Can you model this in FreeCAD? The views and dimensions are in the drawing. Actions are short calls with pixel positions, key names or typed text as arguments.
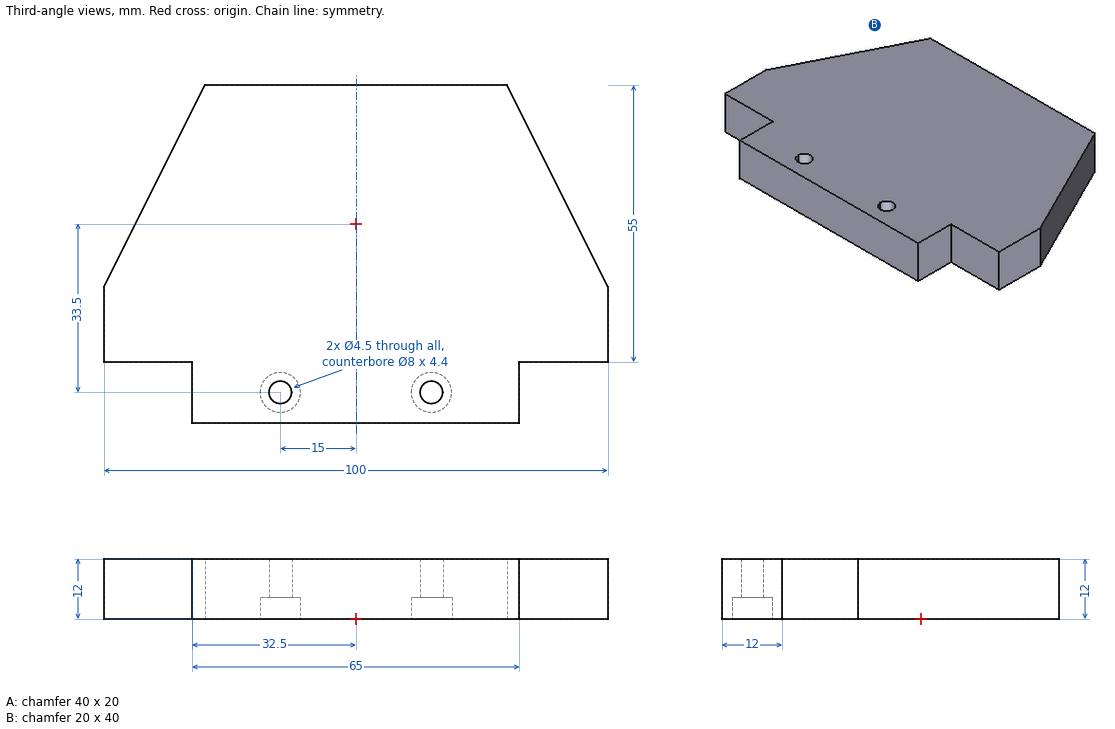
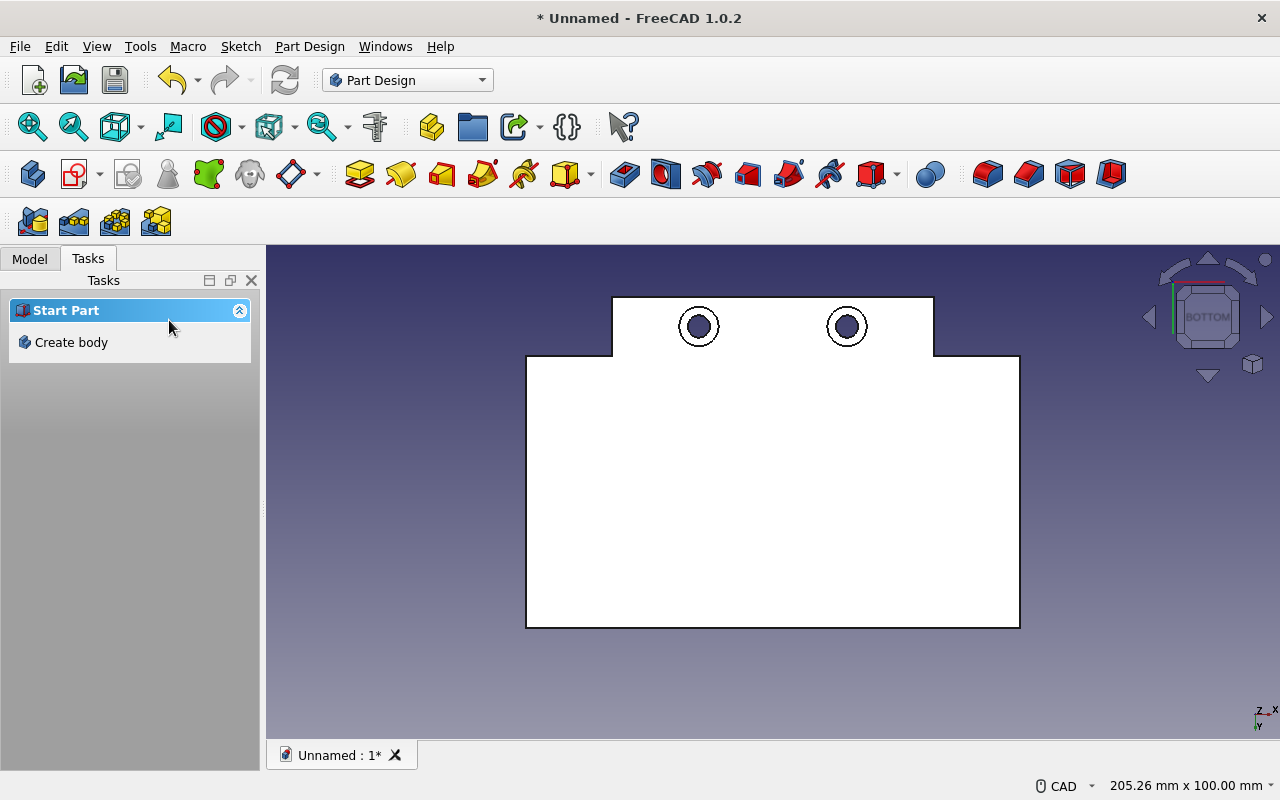
key(0)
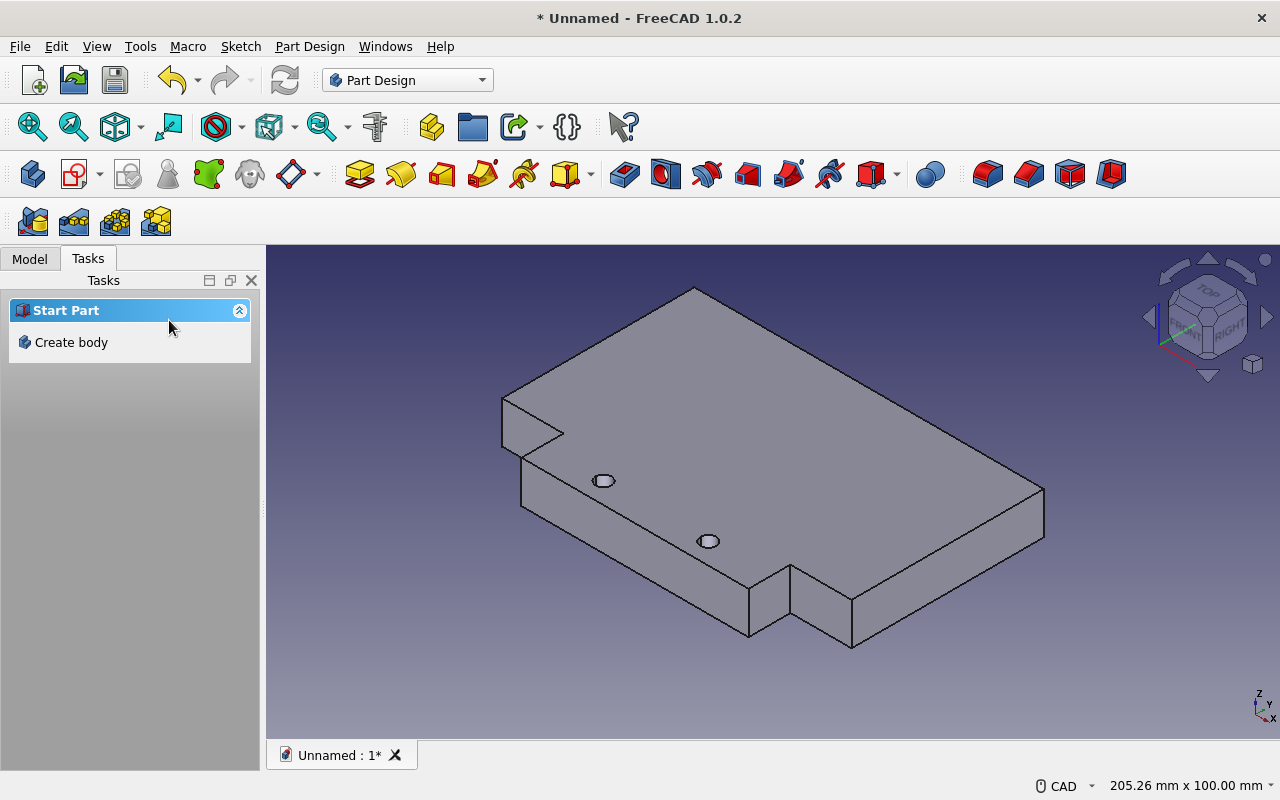
key(2)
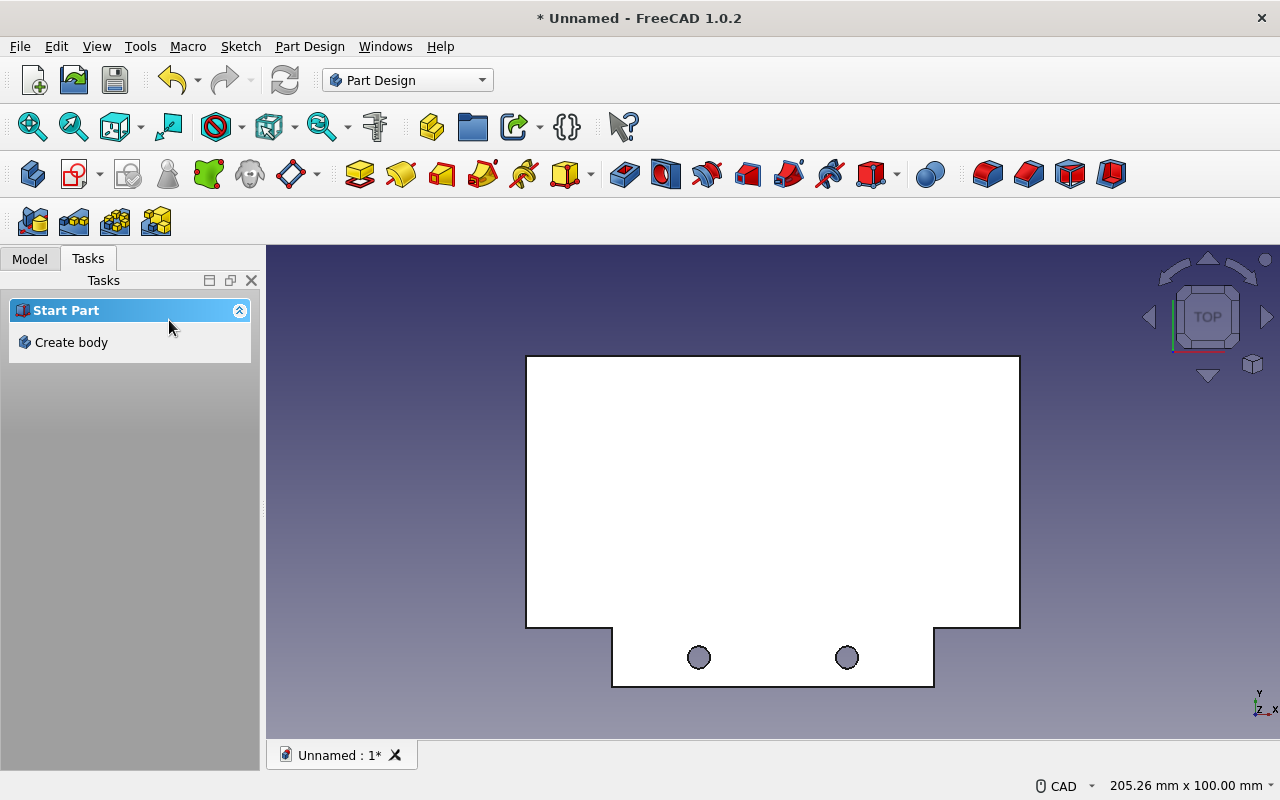
key(1)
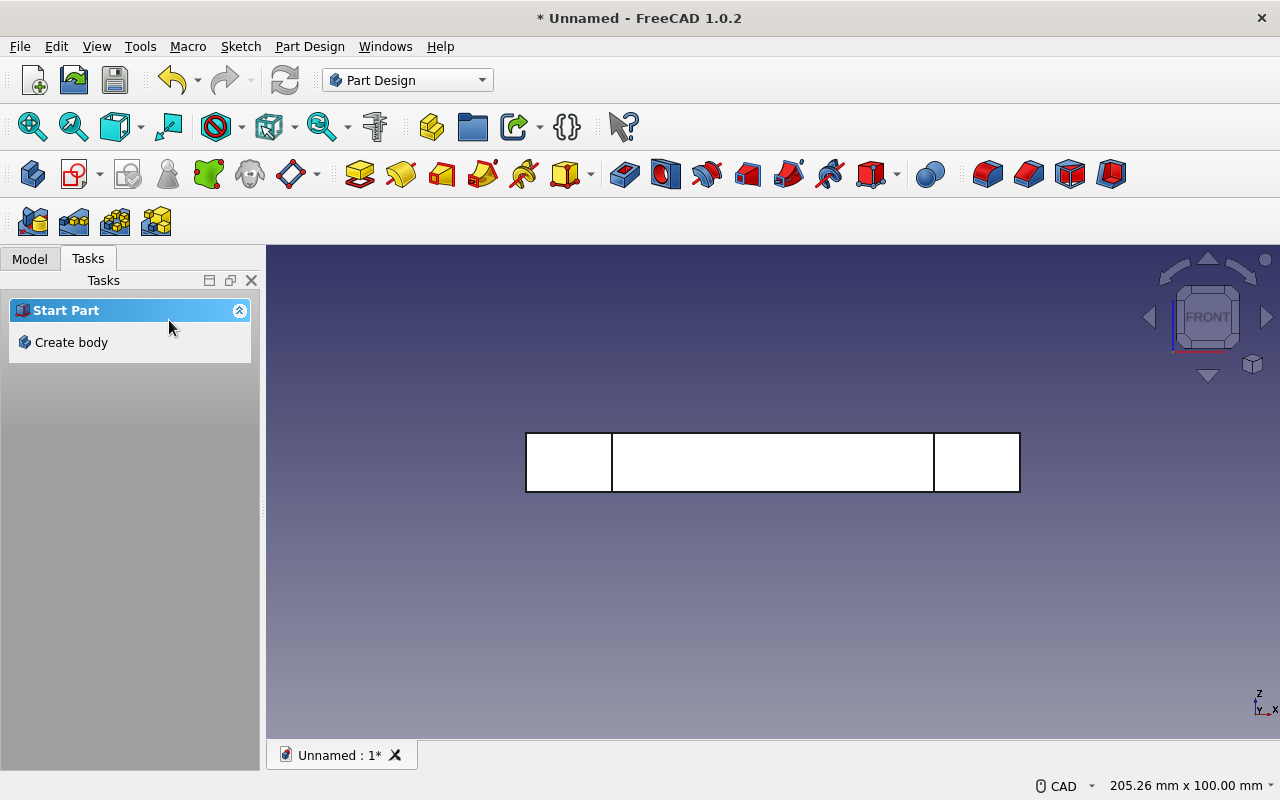
key(3)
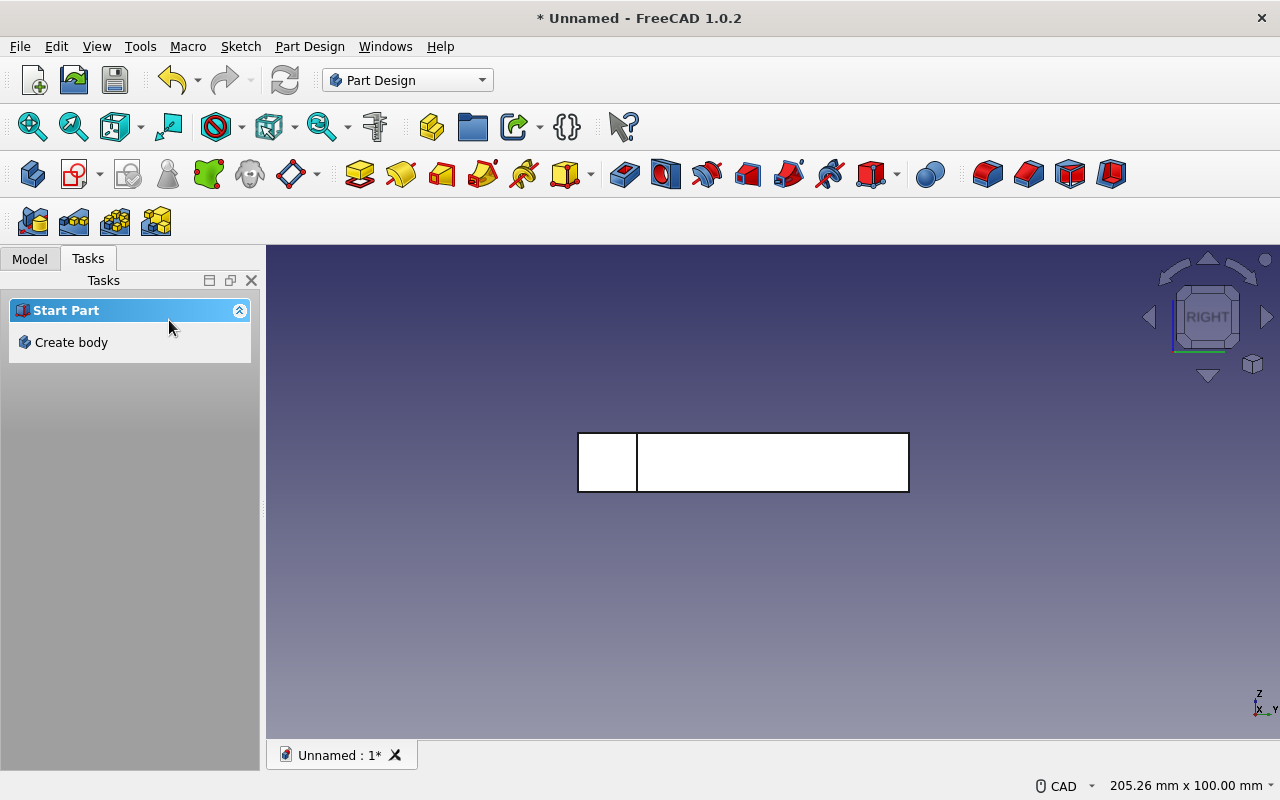
click(33, 128)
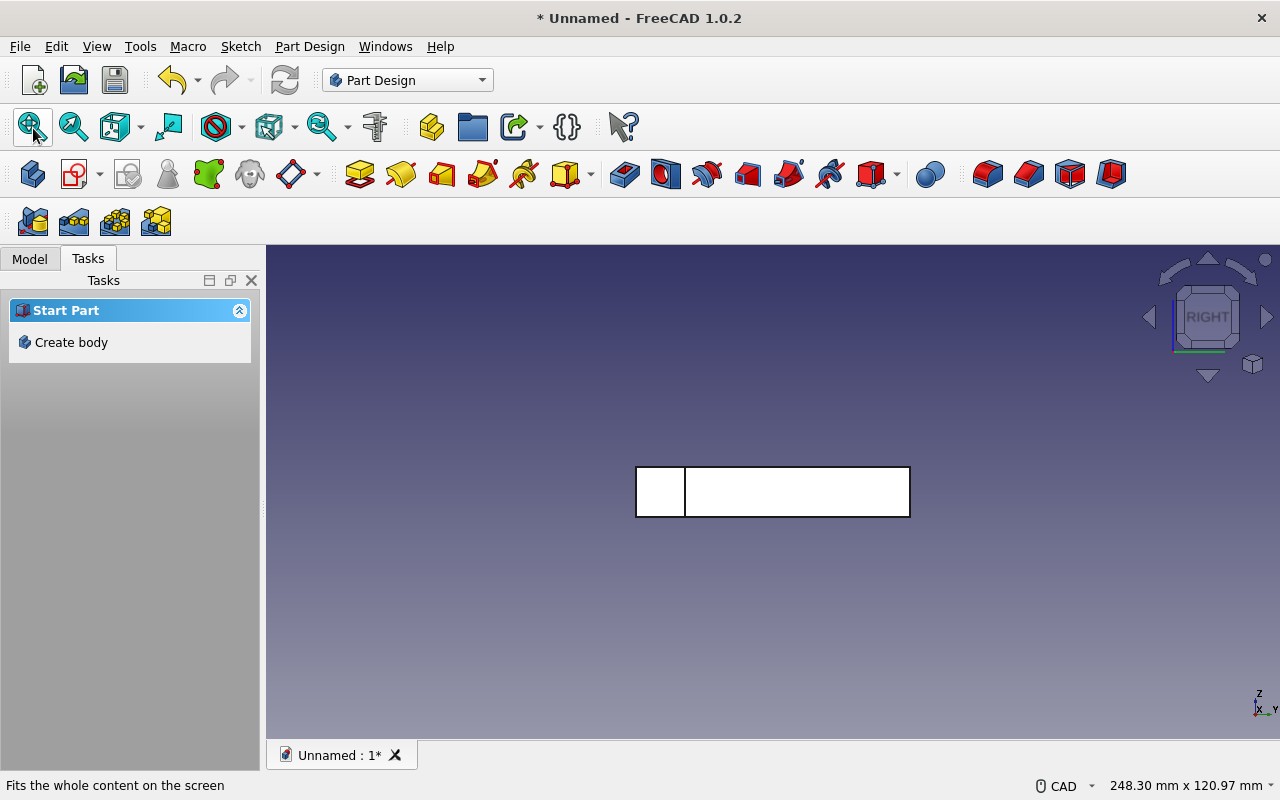
click(910, 491)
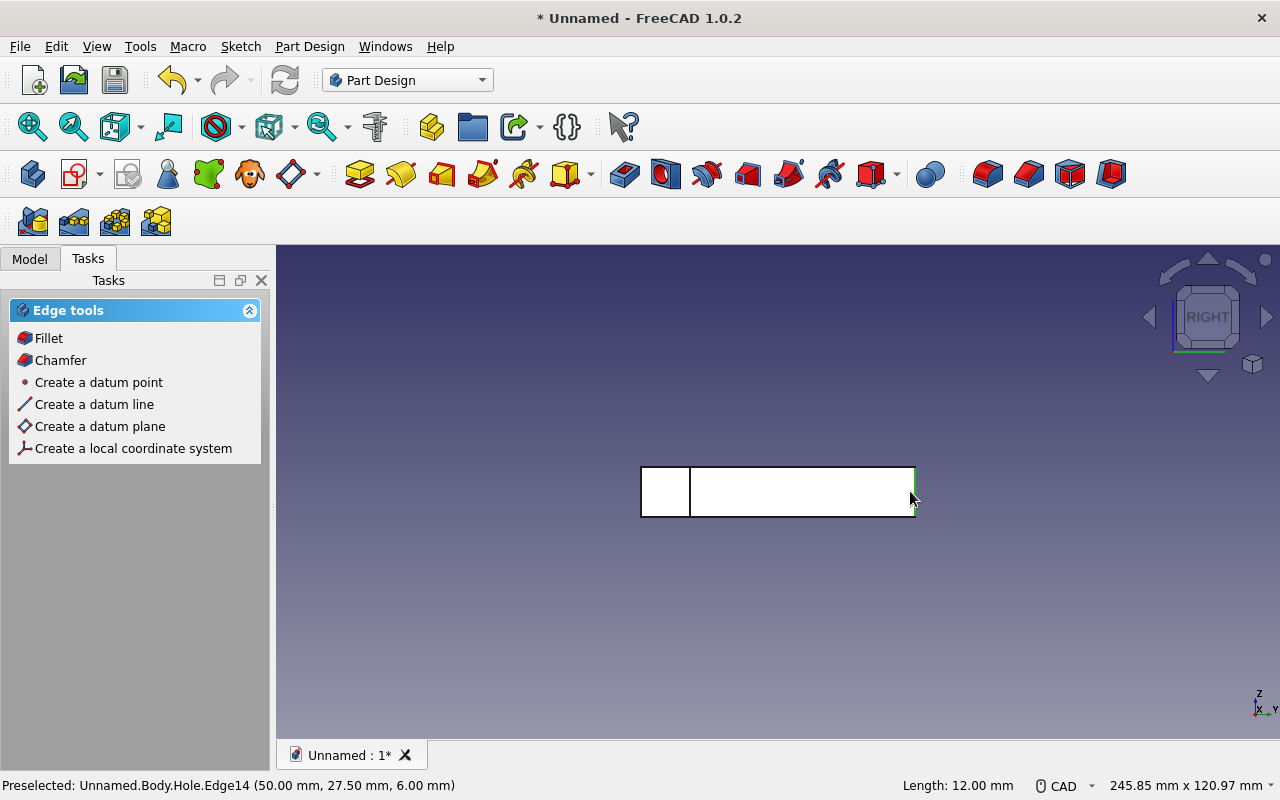
click(1029, 174)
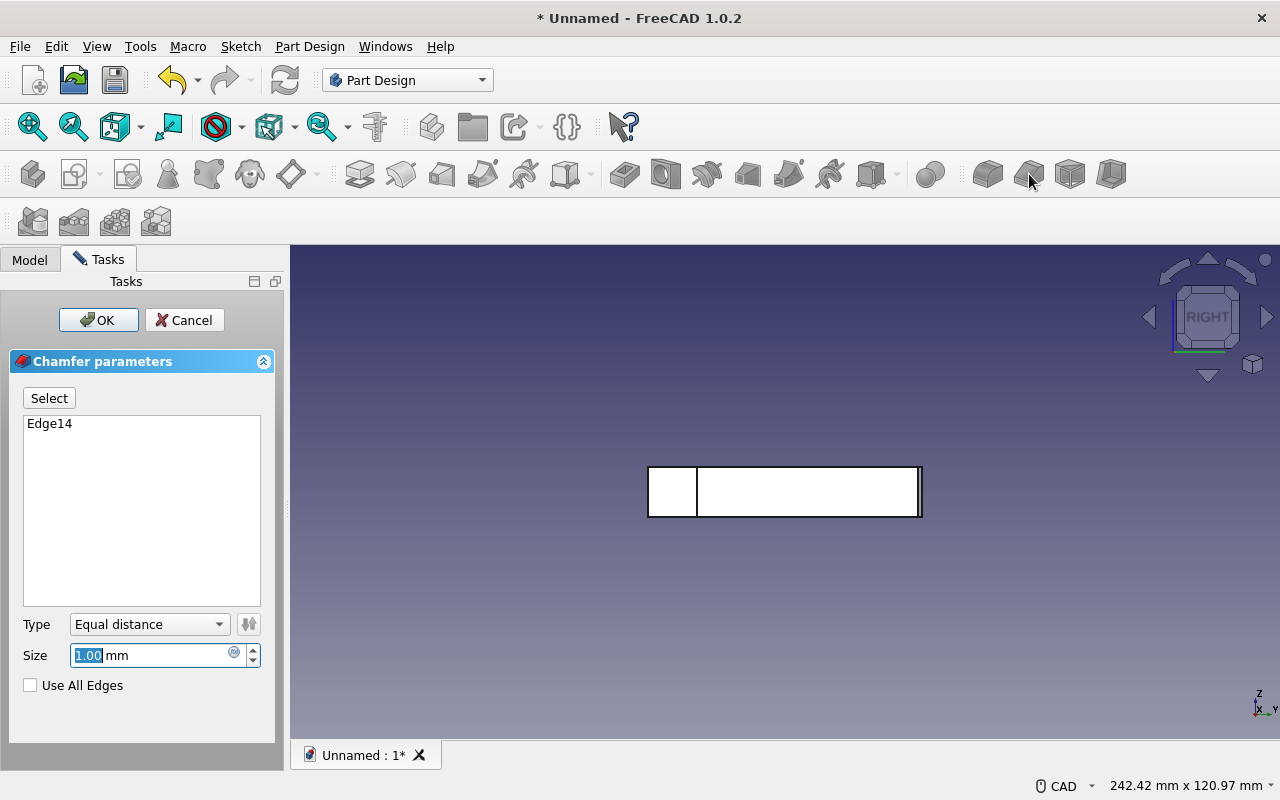
text(40)
key(Tab)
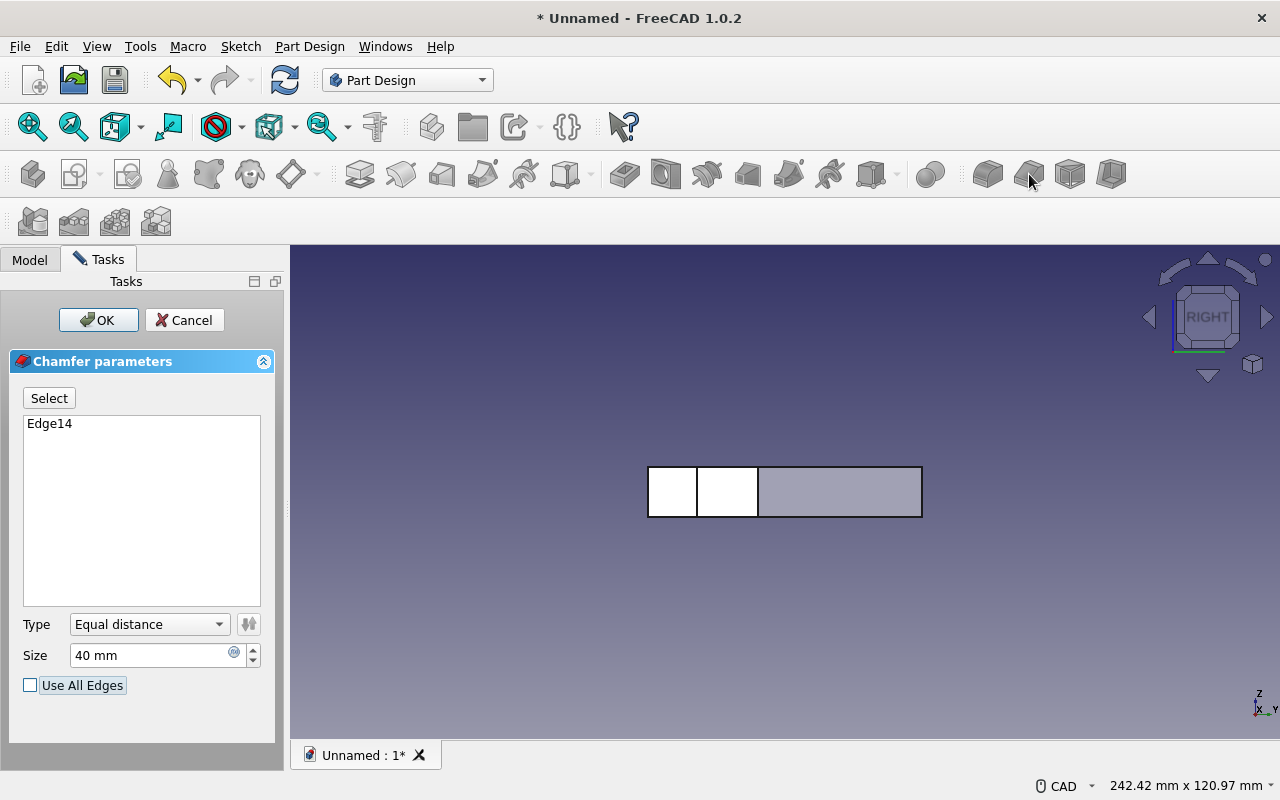
click(150, 624)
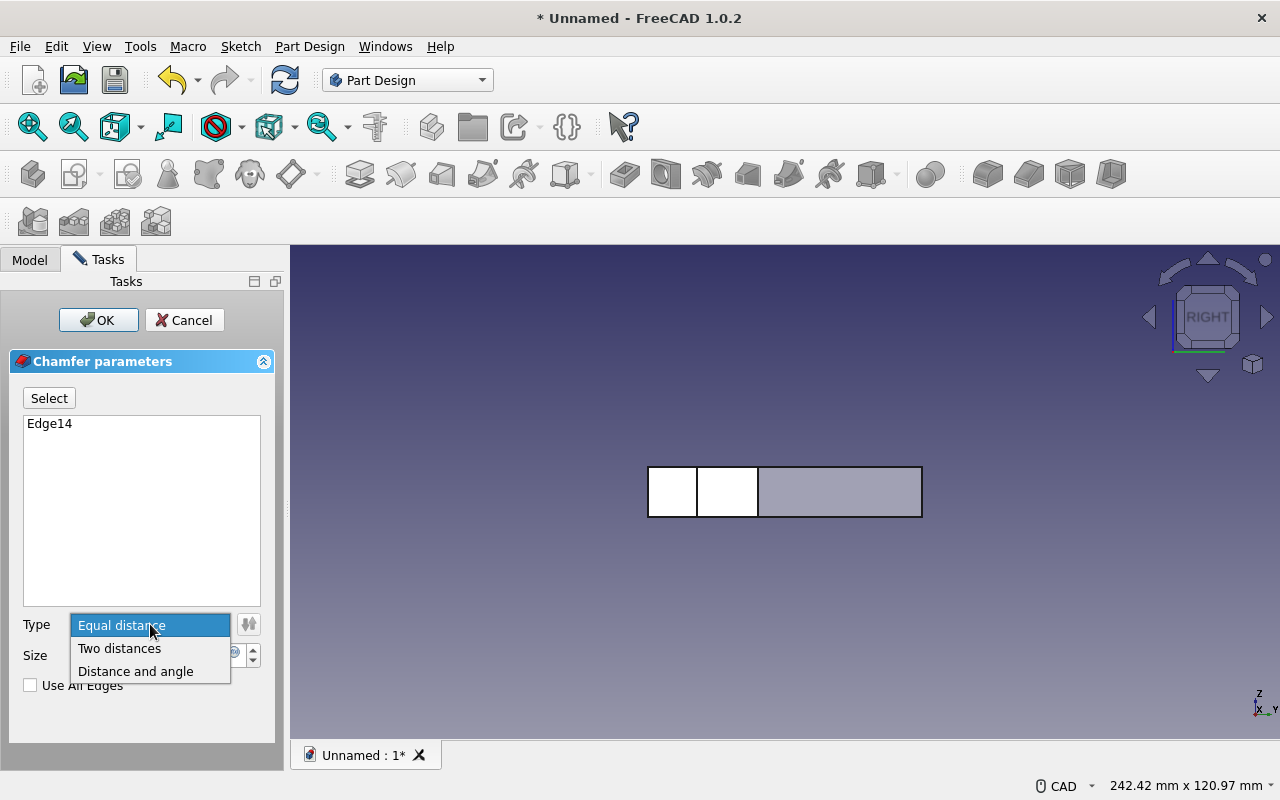
click(148, 648)